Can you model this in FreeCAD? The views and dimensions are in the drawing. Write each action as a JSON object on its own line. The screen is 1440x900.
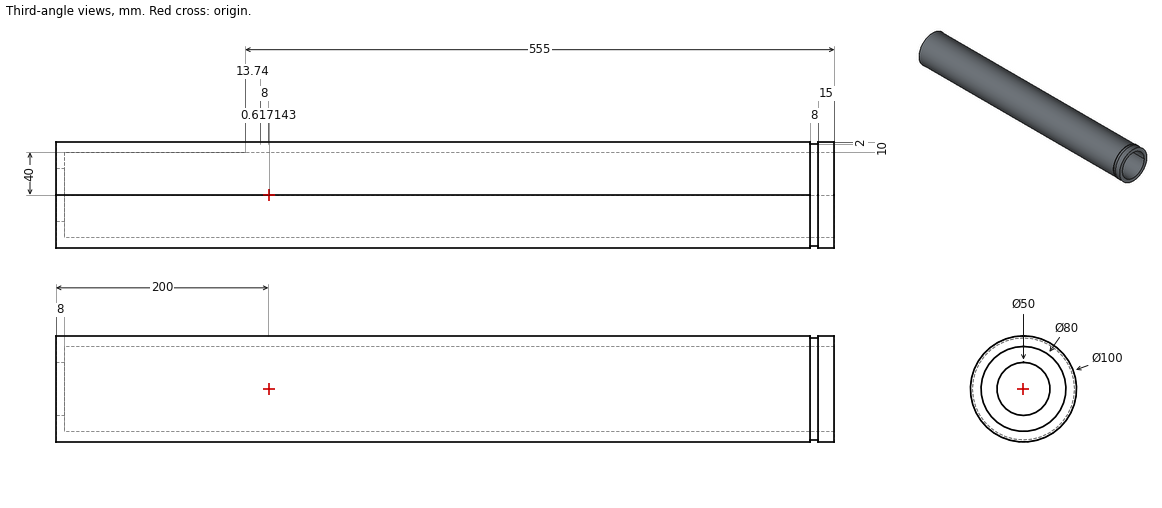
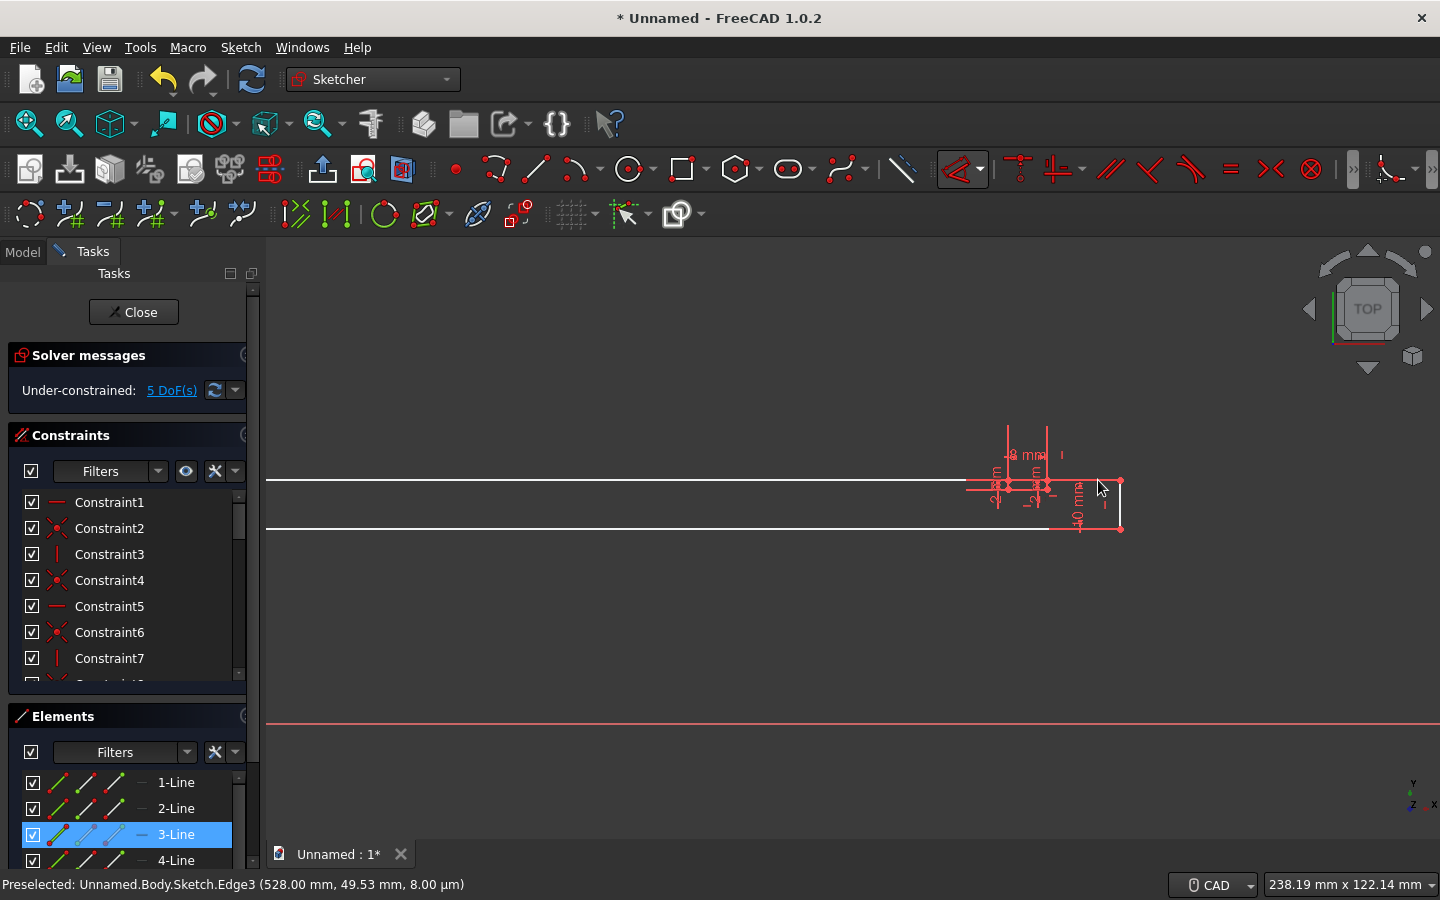
{"action": "key", "text": "l"}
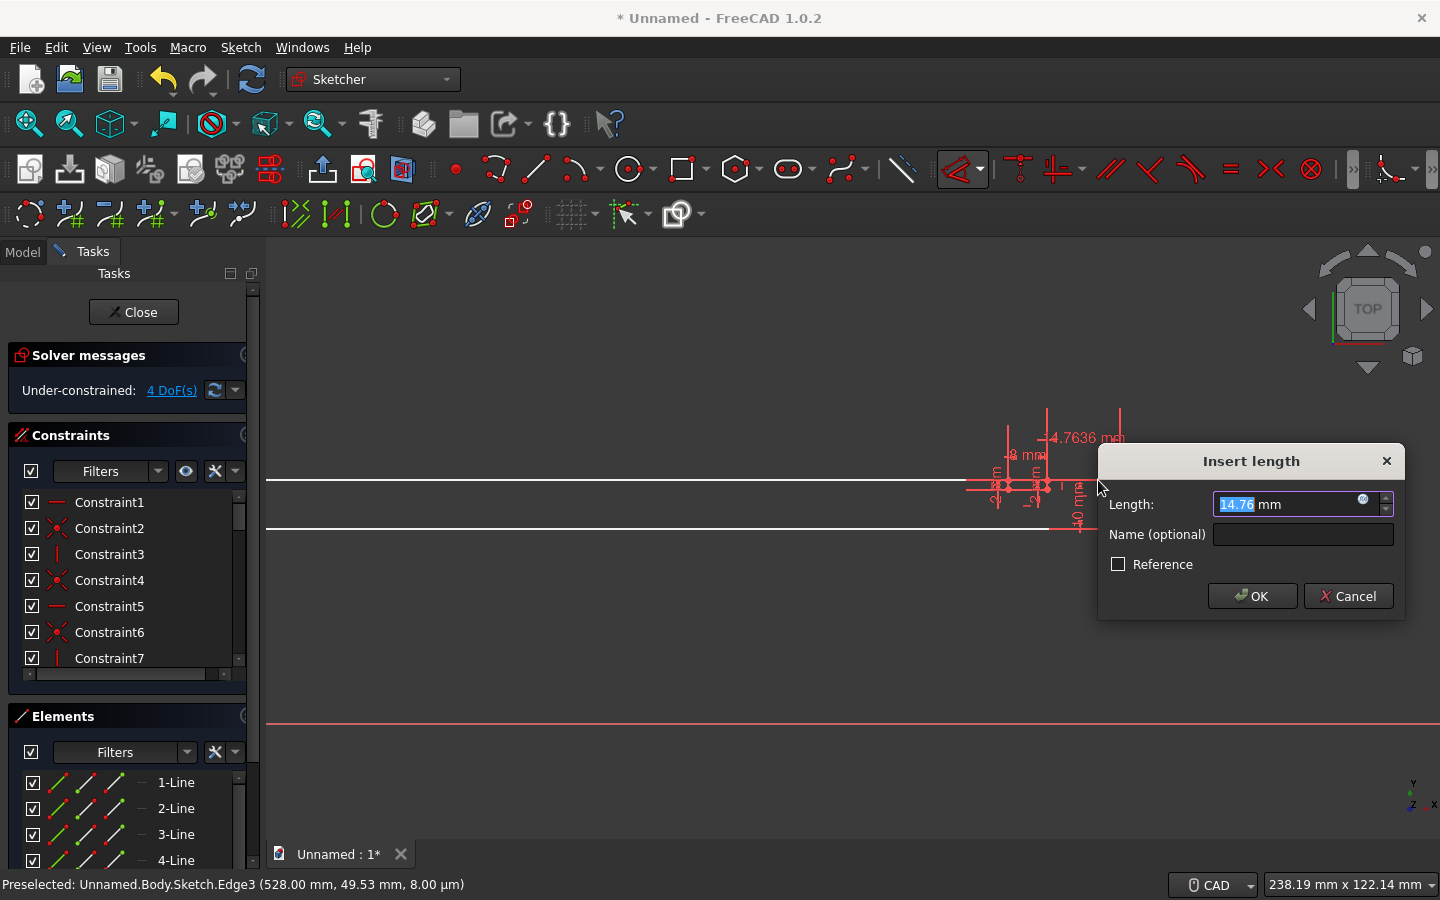
{"action": "type", "text": "15"}
{"action": "key", "text": "Return"}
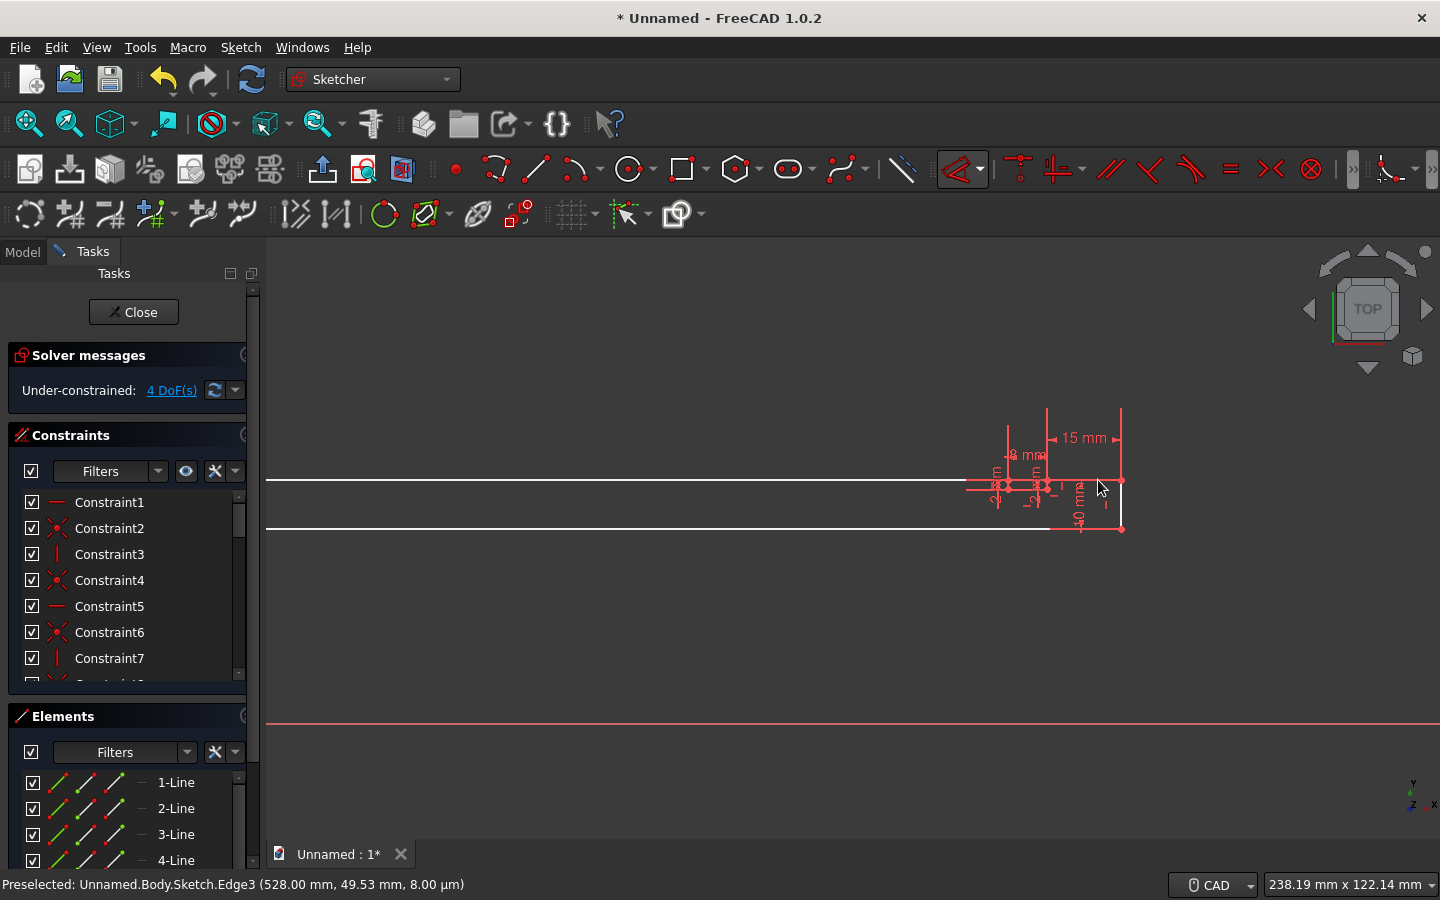
{"action": "scroll", "coordinate": [1122, 517], "scroll_direction": "down", "scroll_amount": 7}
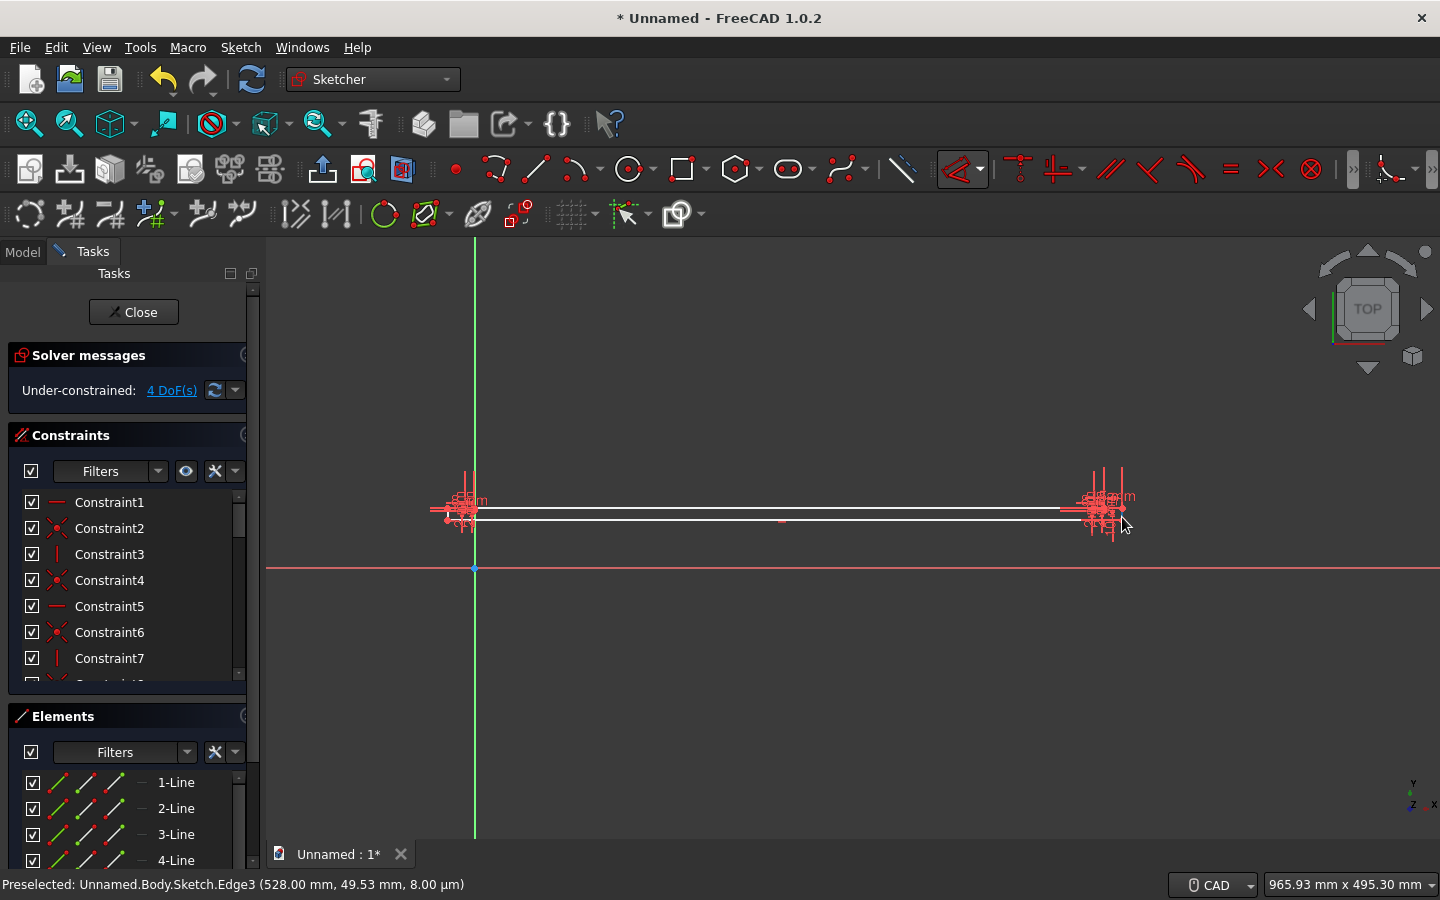
{"action": "left_click", "coordinate": [920, 520]}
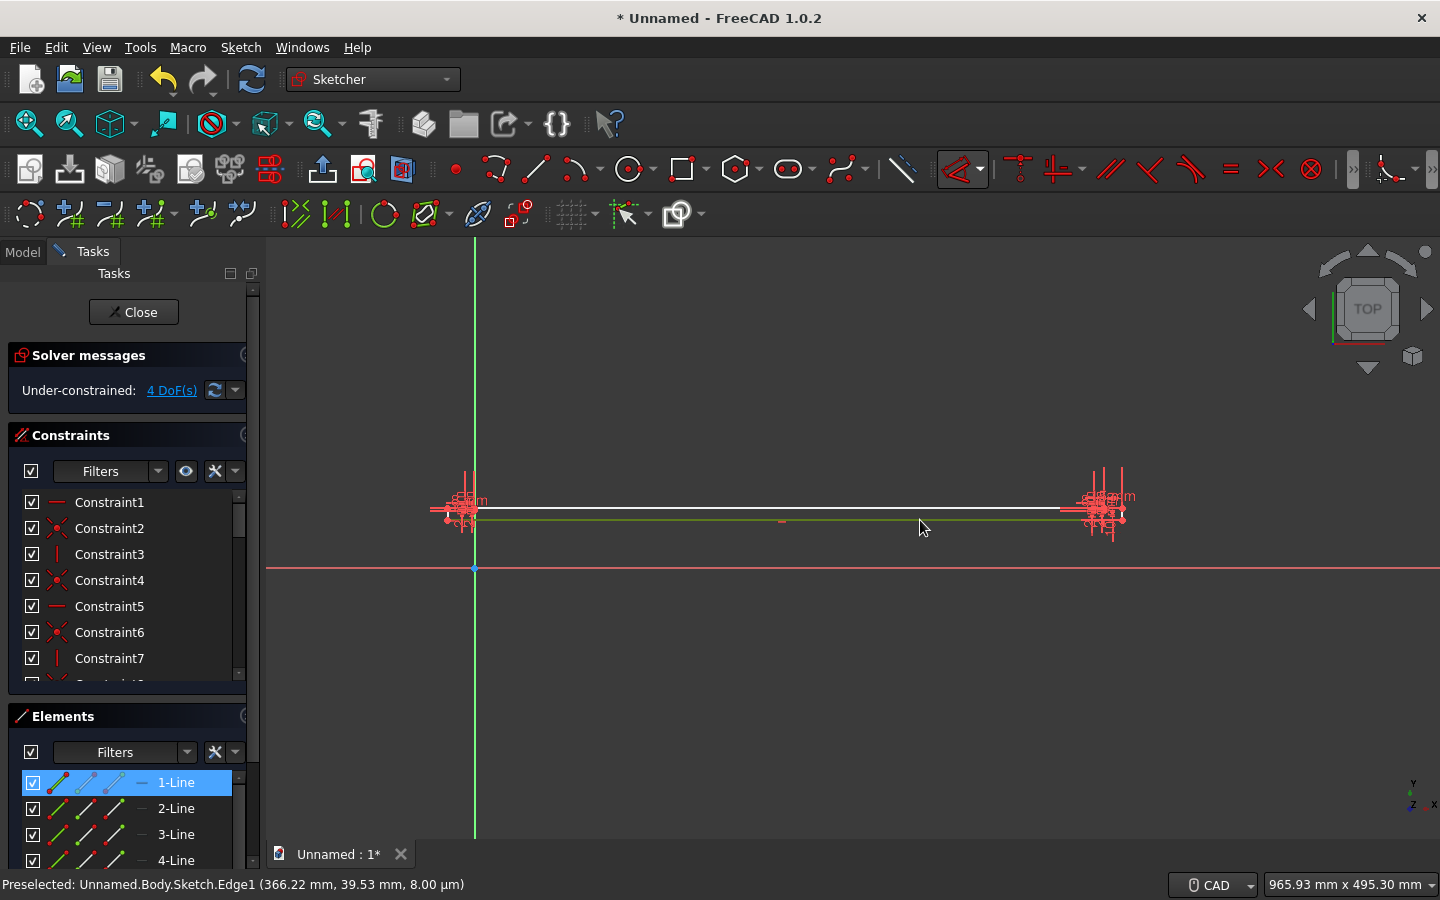
{"action": "left_click", "coordinate": [982, 170]}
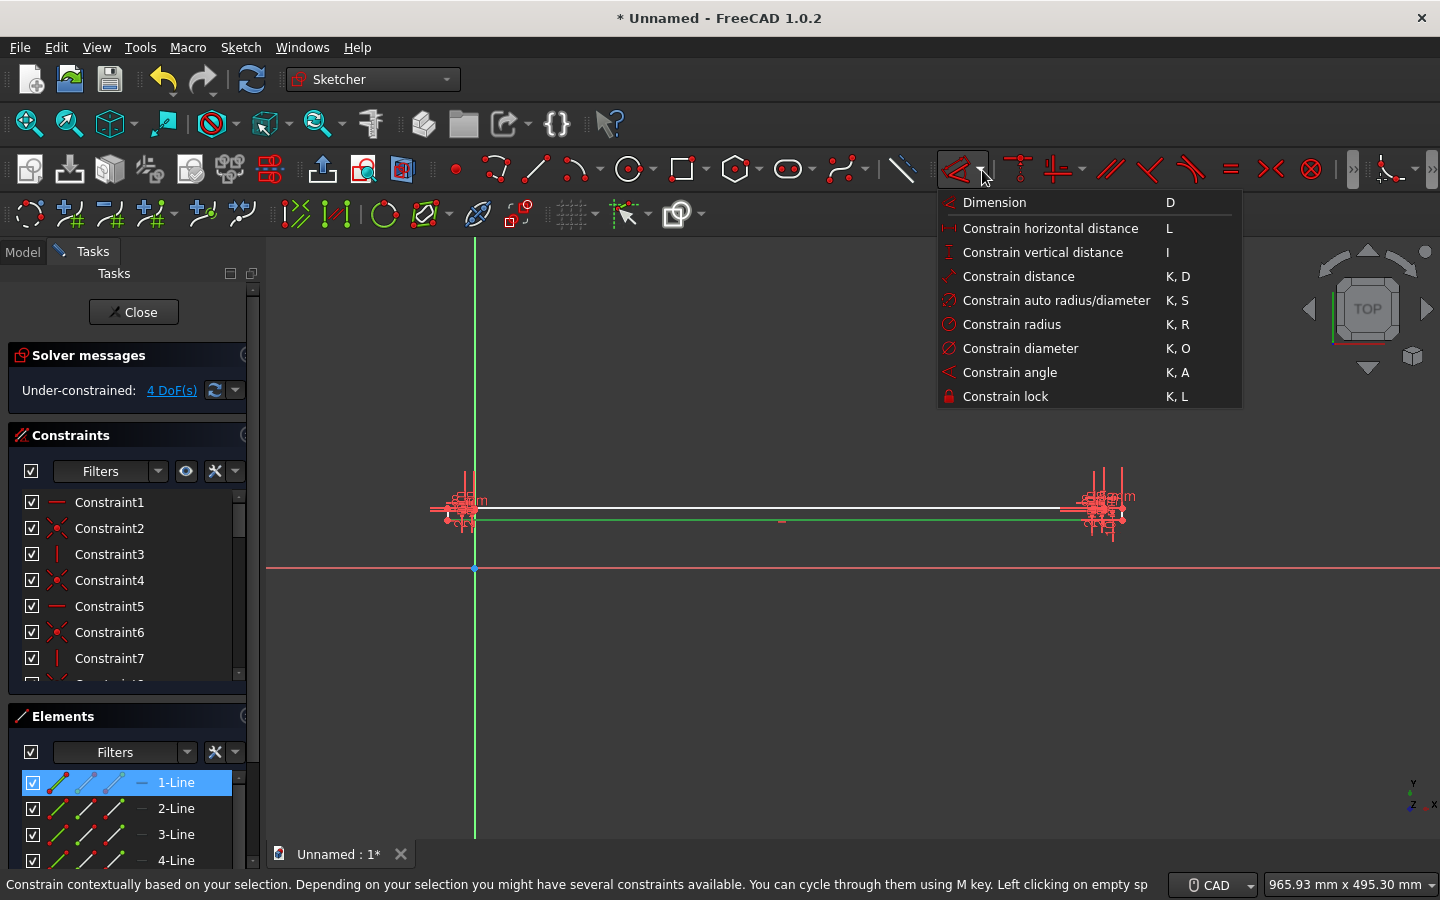
{"action": "left_click", "coordinate": [1090, 228]}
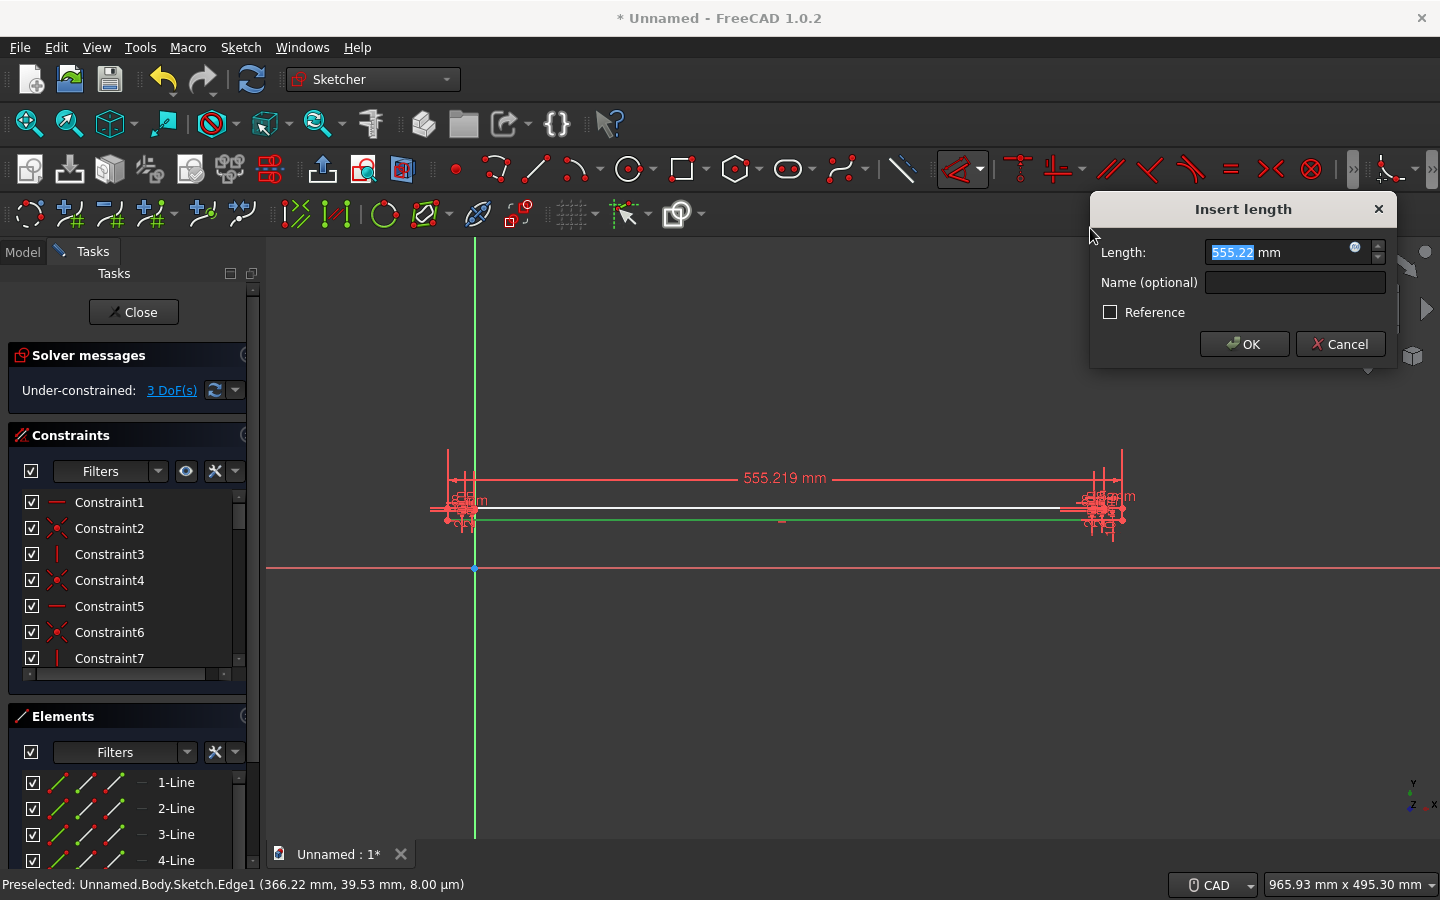
{"action": "type", "text": "555"}
{"action": "key", "text": "Return"}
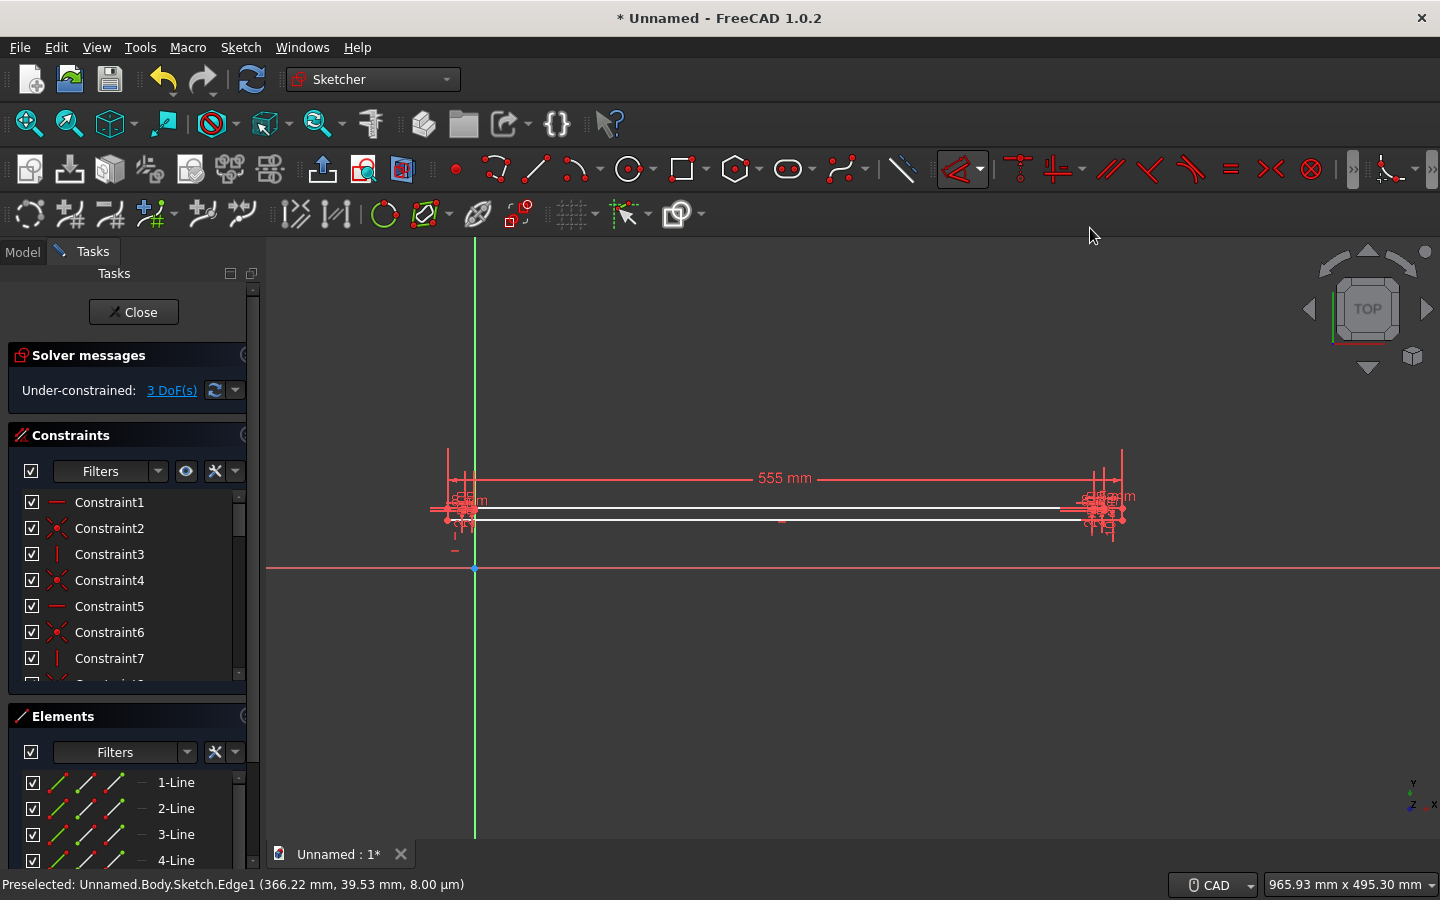
{"action": "left_click", "coordinate": [448, 520]}